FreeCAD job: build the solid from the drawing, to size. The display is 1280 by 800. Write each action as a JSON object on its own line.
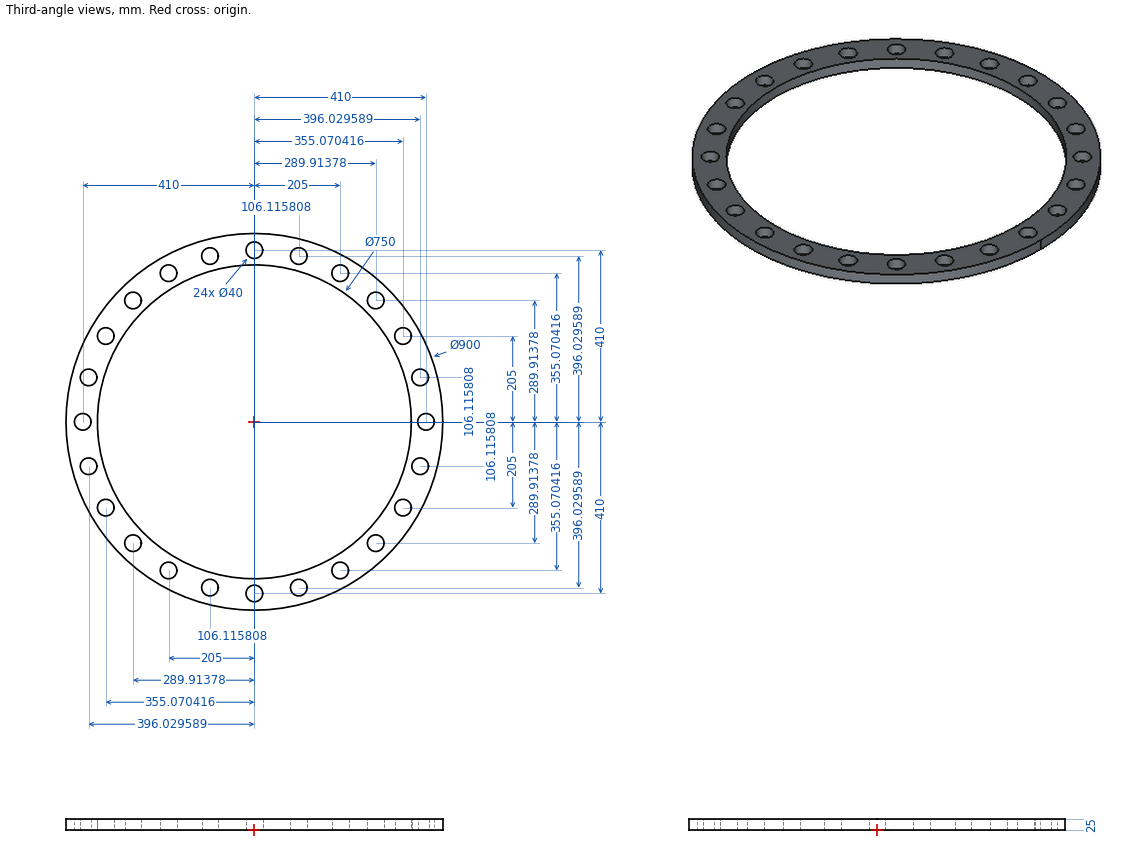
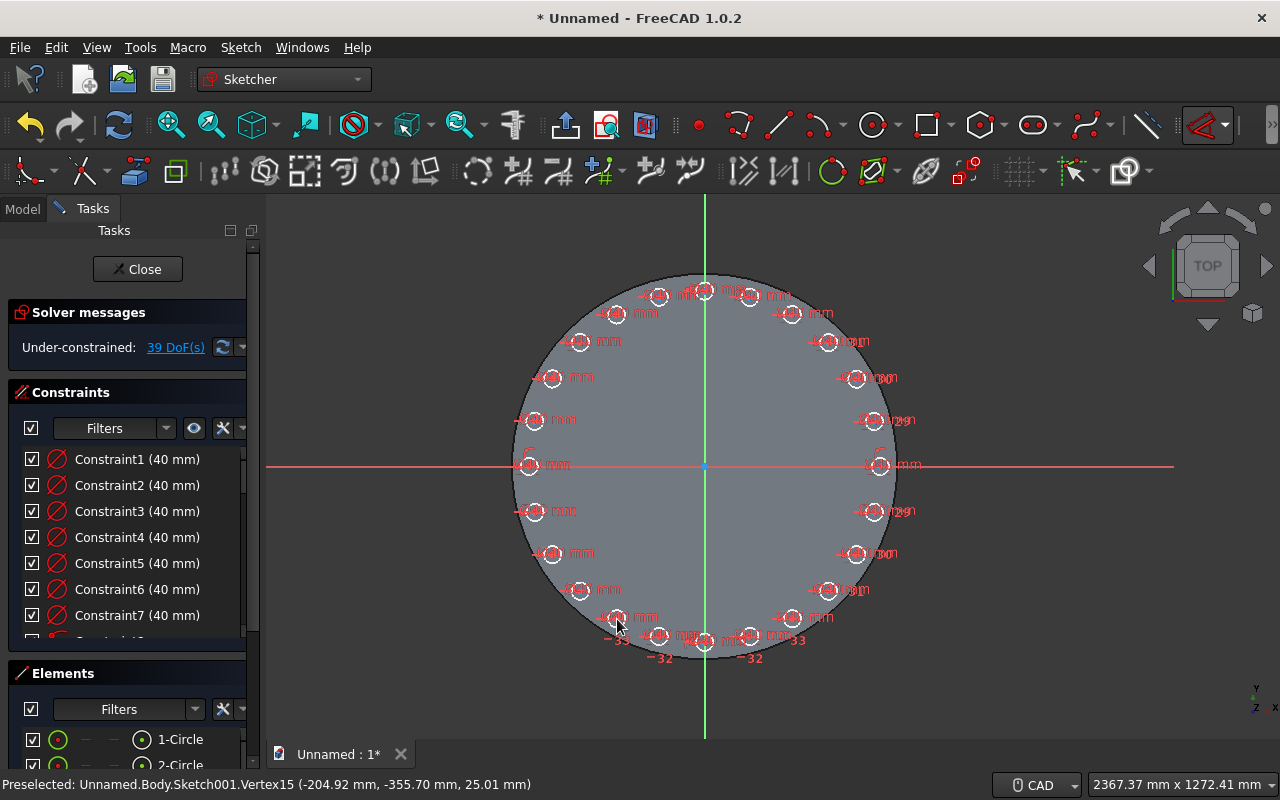
{"action": "left_click", "coordinate": [829, 591]}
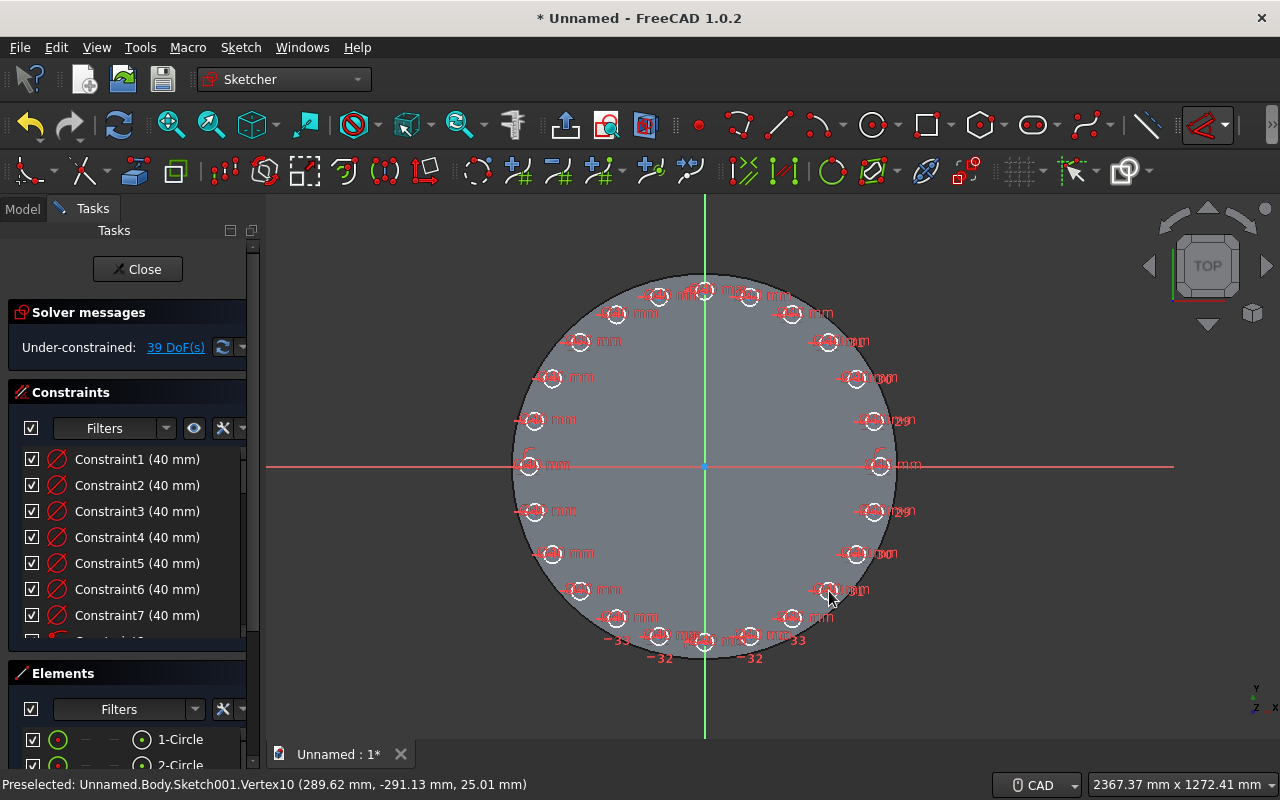
{"action": "left_click", "coordinate": [580, 591]}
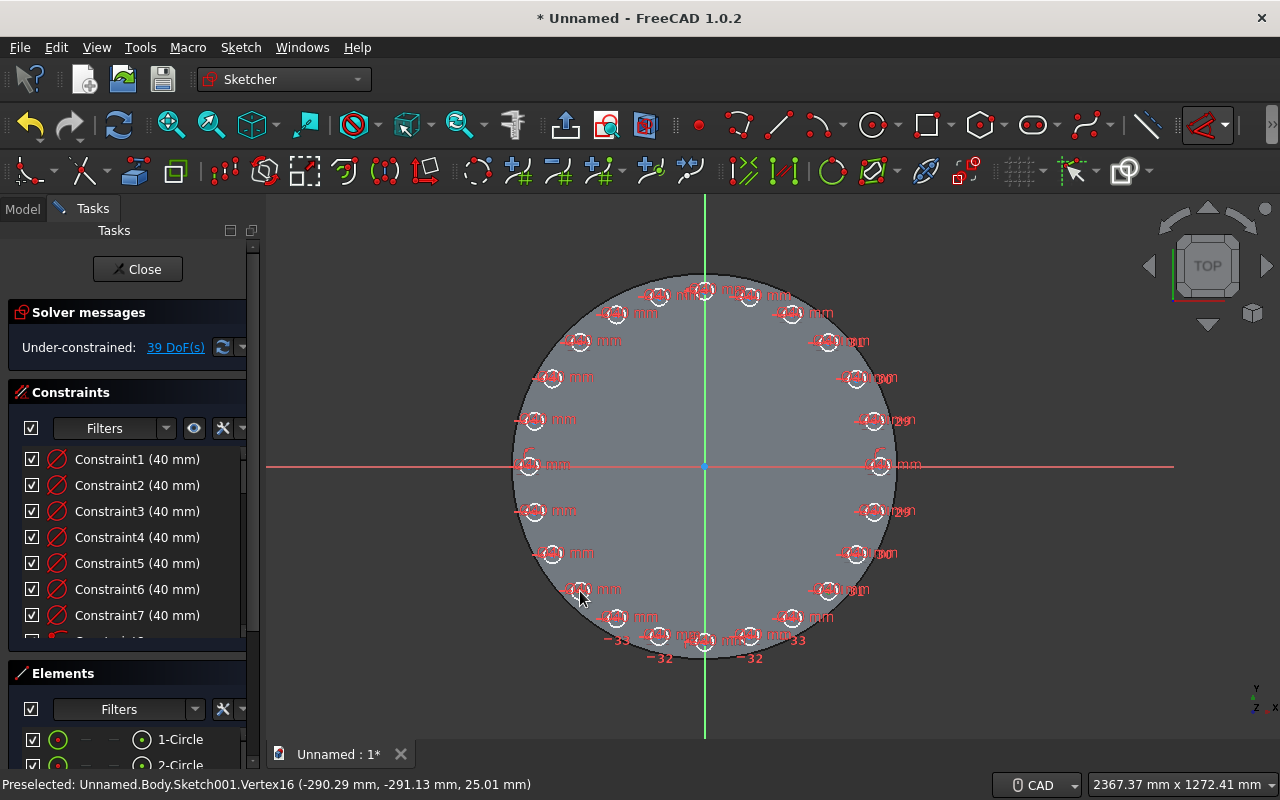
{"action": "key", "text": "h"}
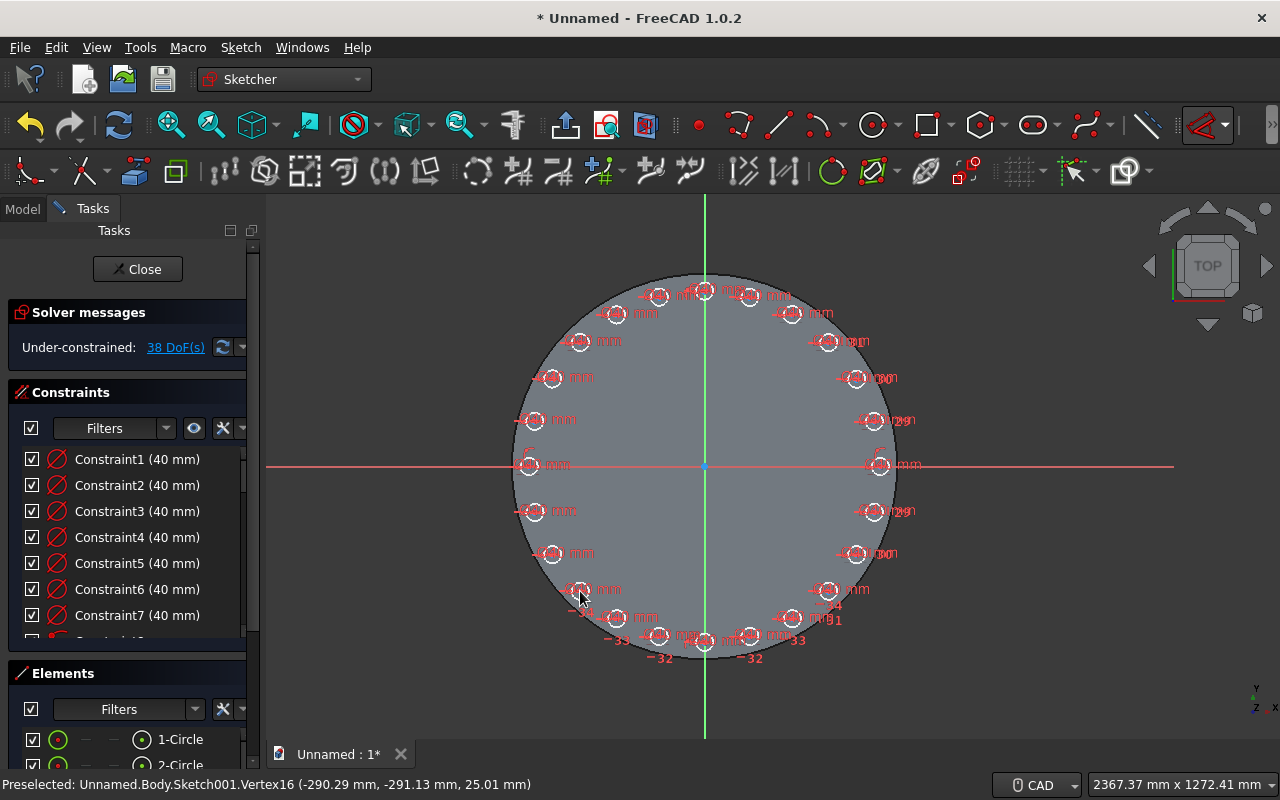
{"action": "left_click", "coordinate": [535, 512]}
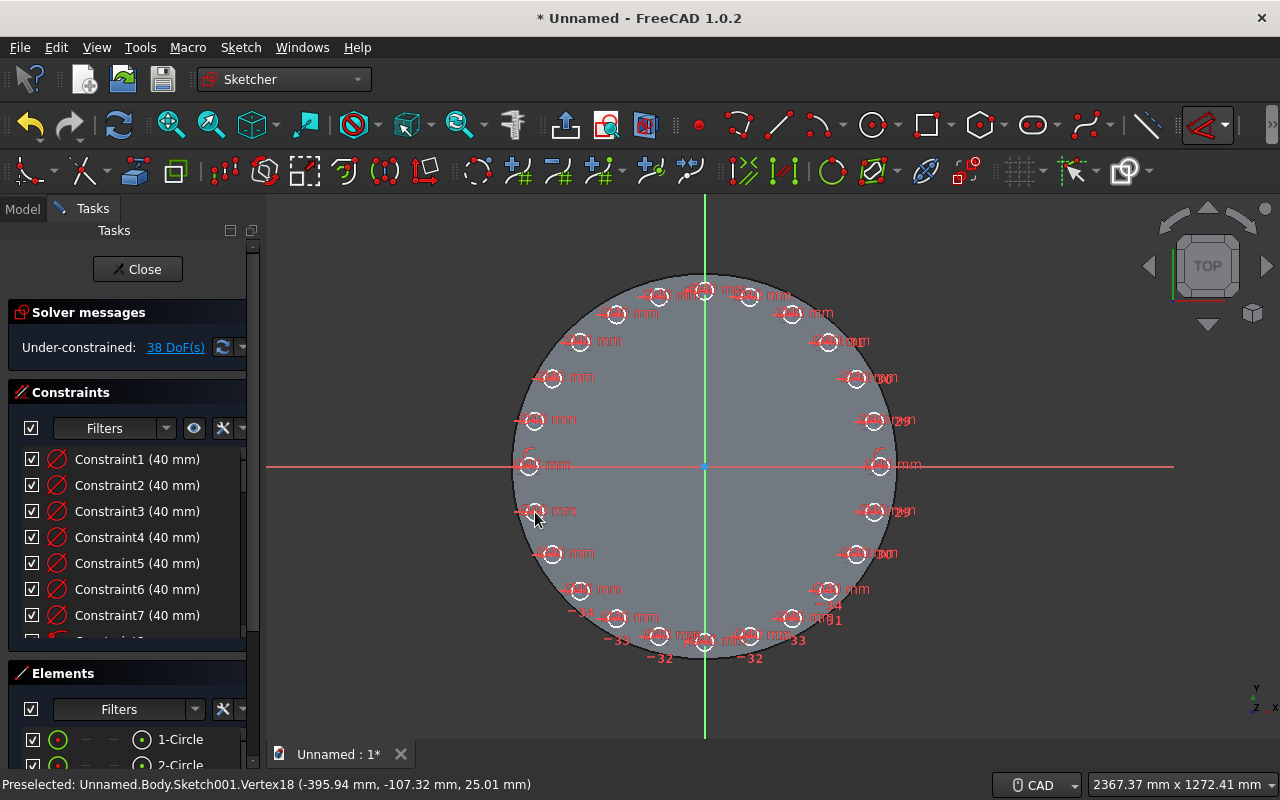
{"action": "left_click", "coordinate": [535, 421]}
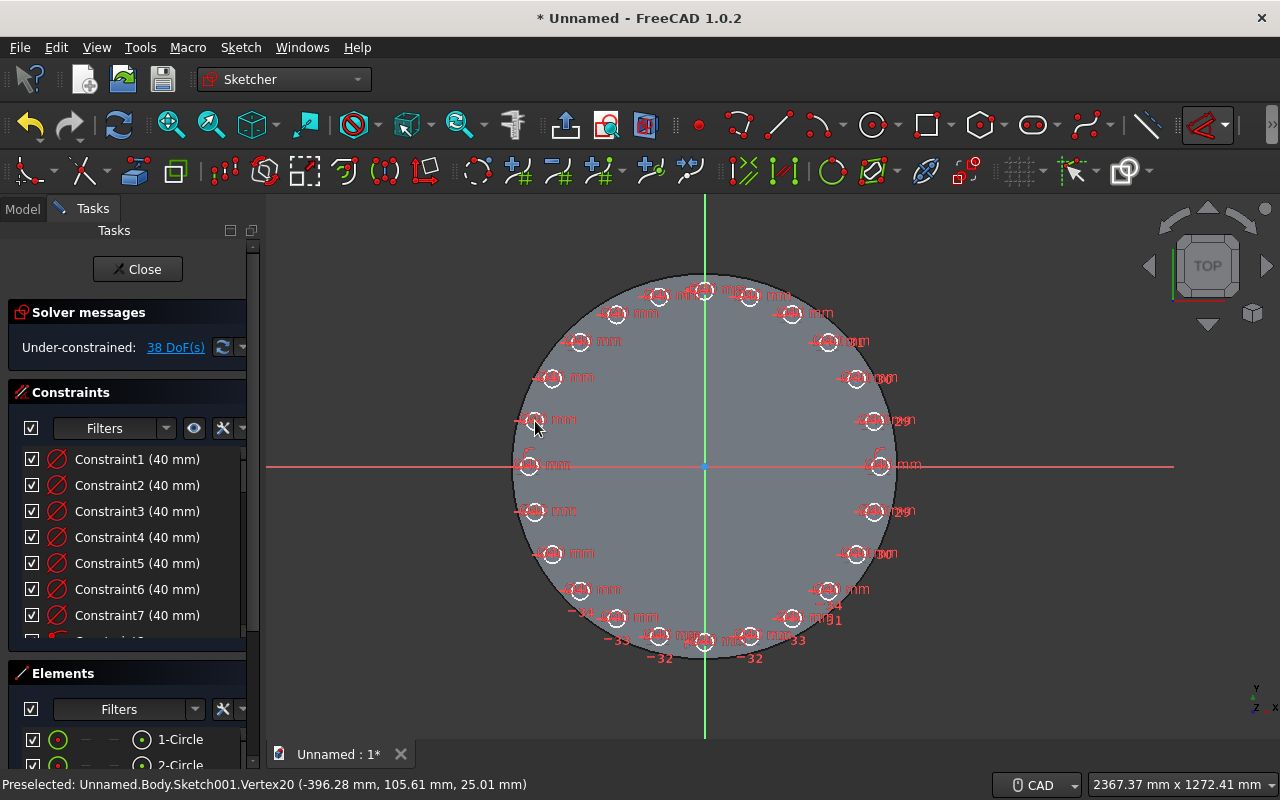
{"action": "key", "text": "v"}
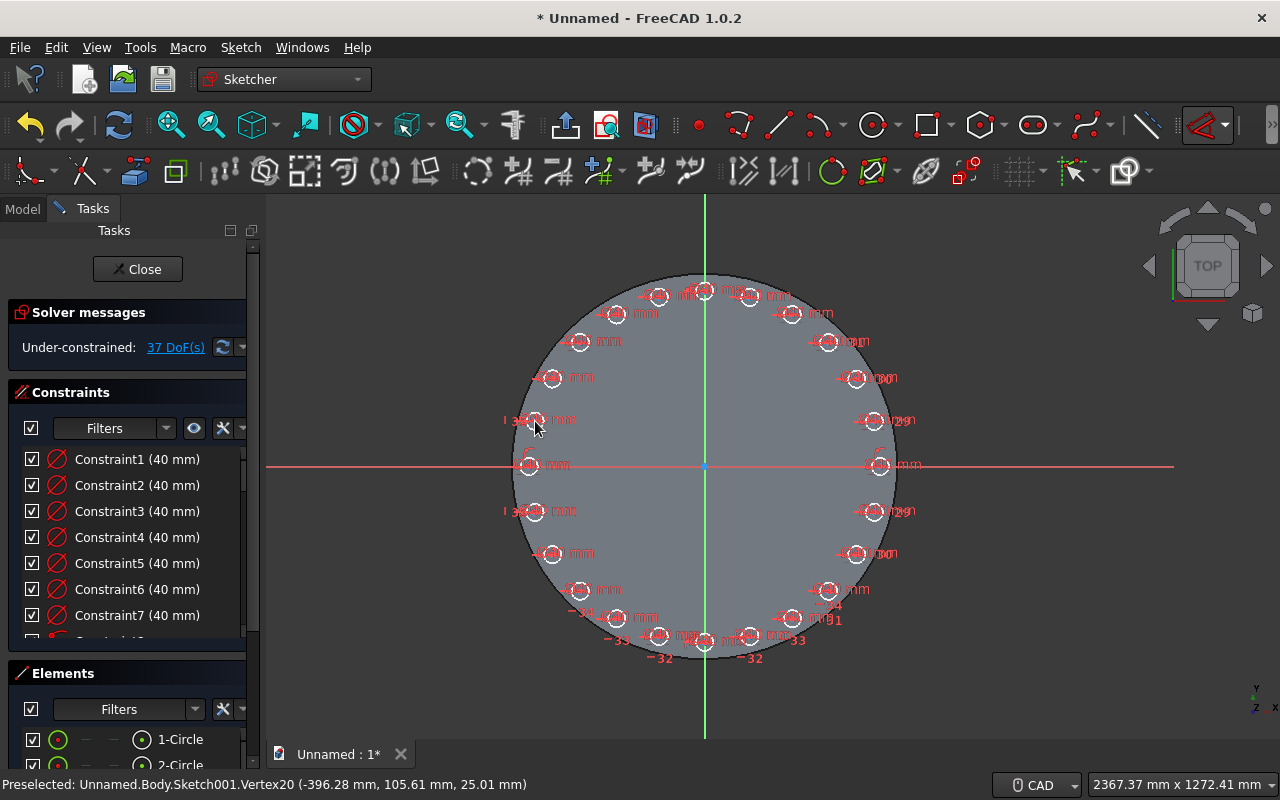
{"action": "left_click", "coordinate": [553, 555]}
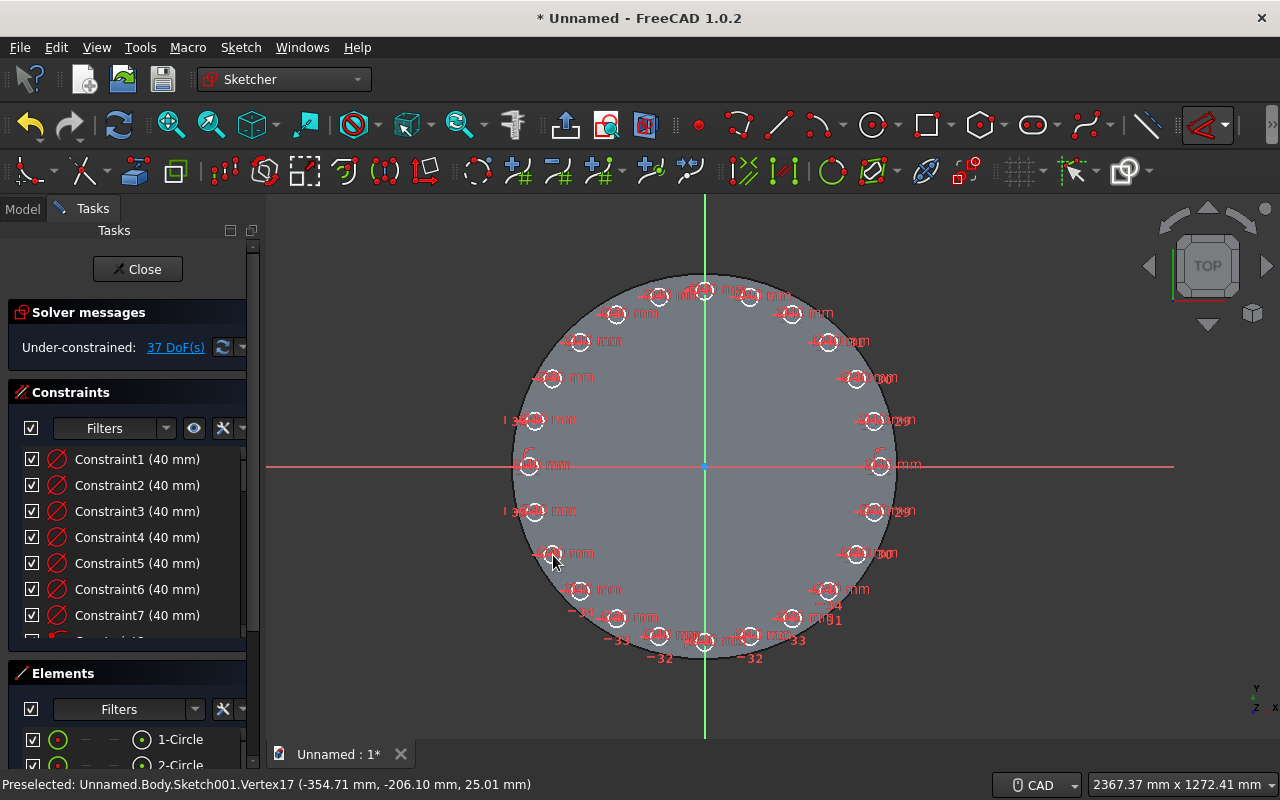
{"action": "left_click", "coordinate": [552, 379]}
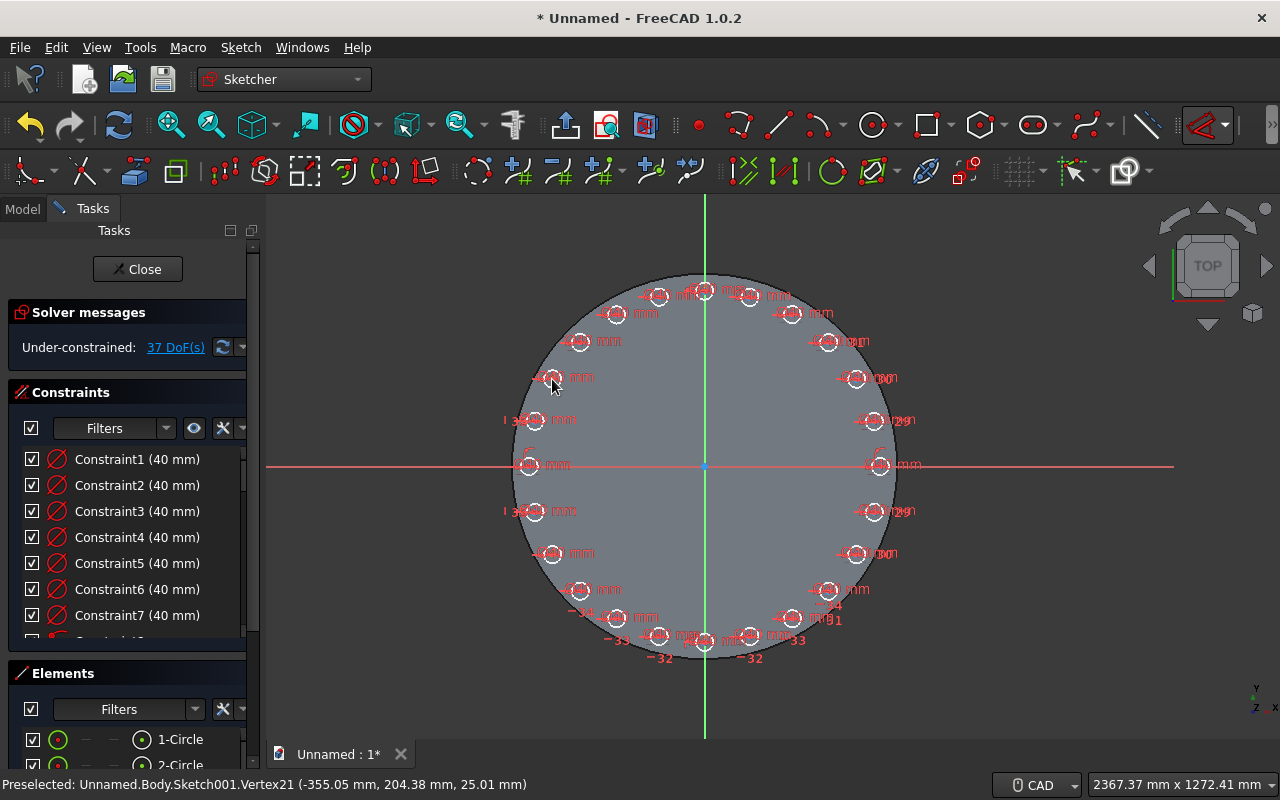
{"action": "key", "text": "v"}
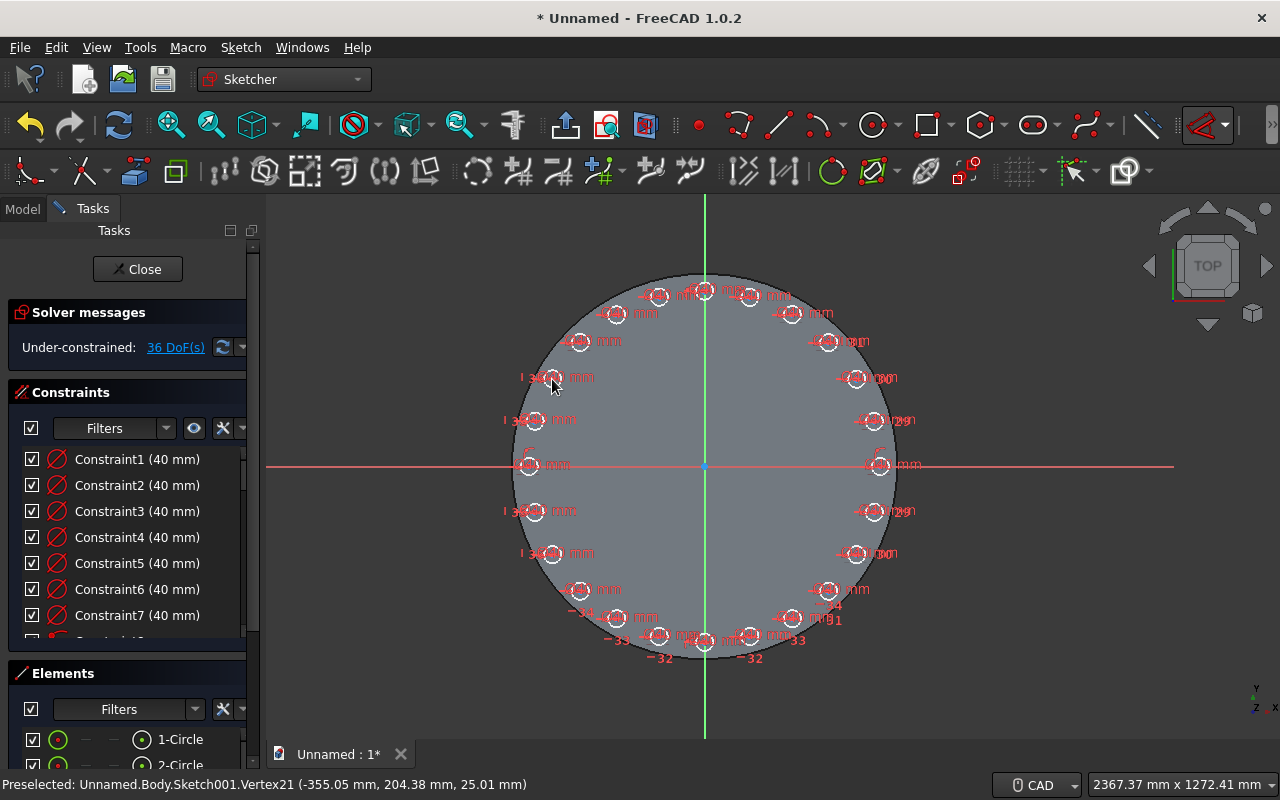
{"action": "left_click", "coordinate": [792, 315]}